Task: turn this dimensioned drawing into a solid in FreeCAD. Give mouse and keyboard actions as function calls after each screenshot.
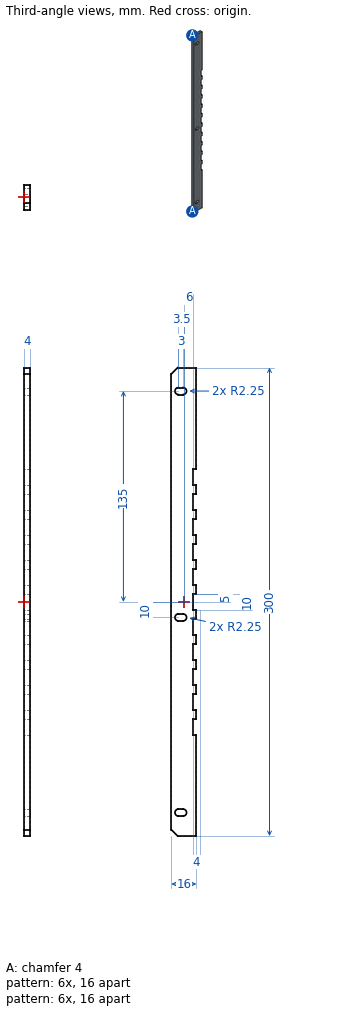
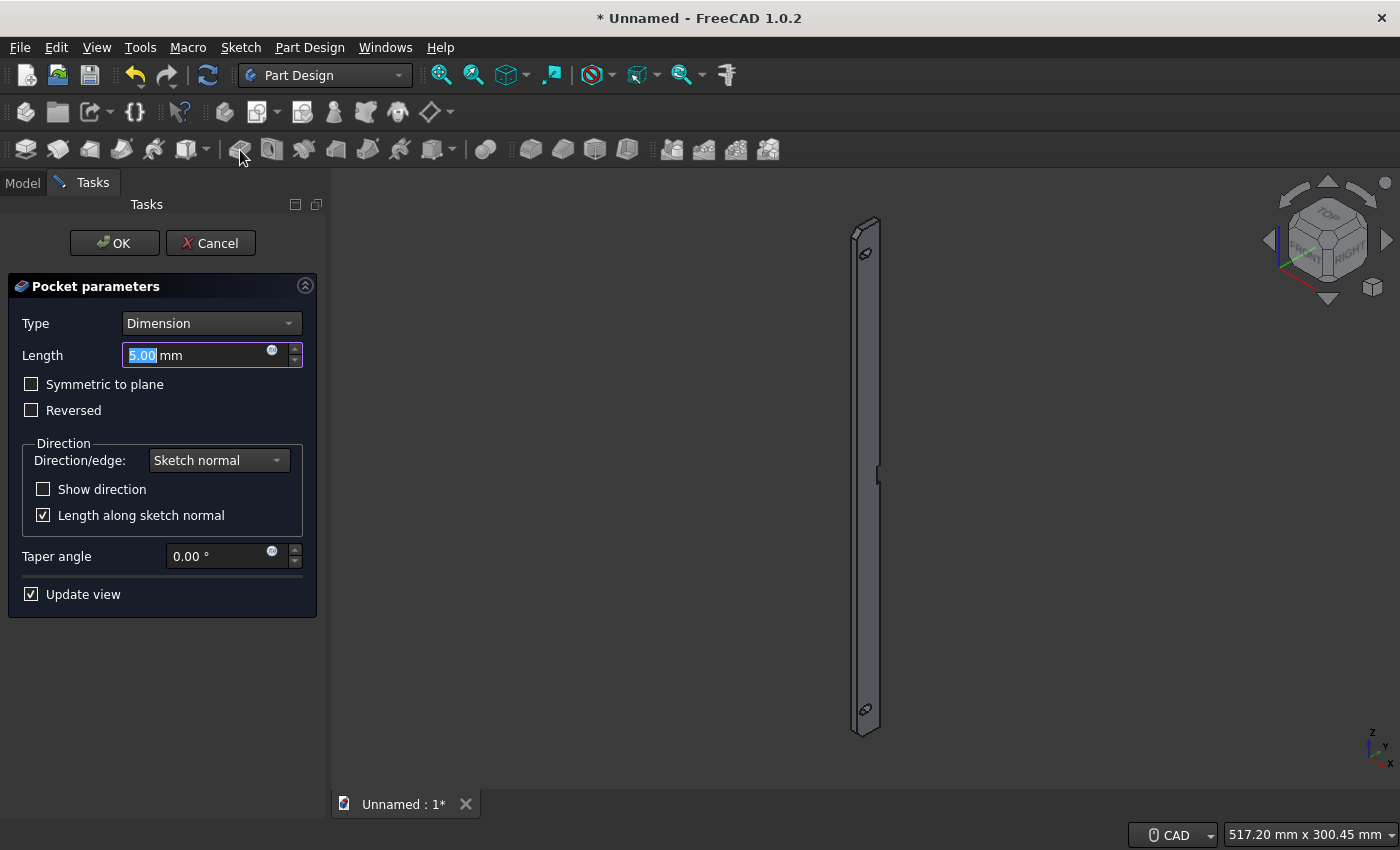
click(212, 324)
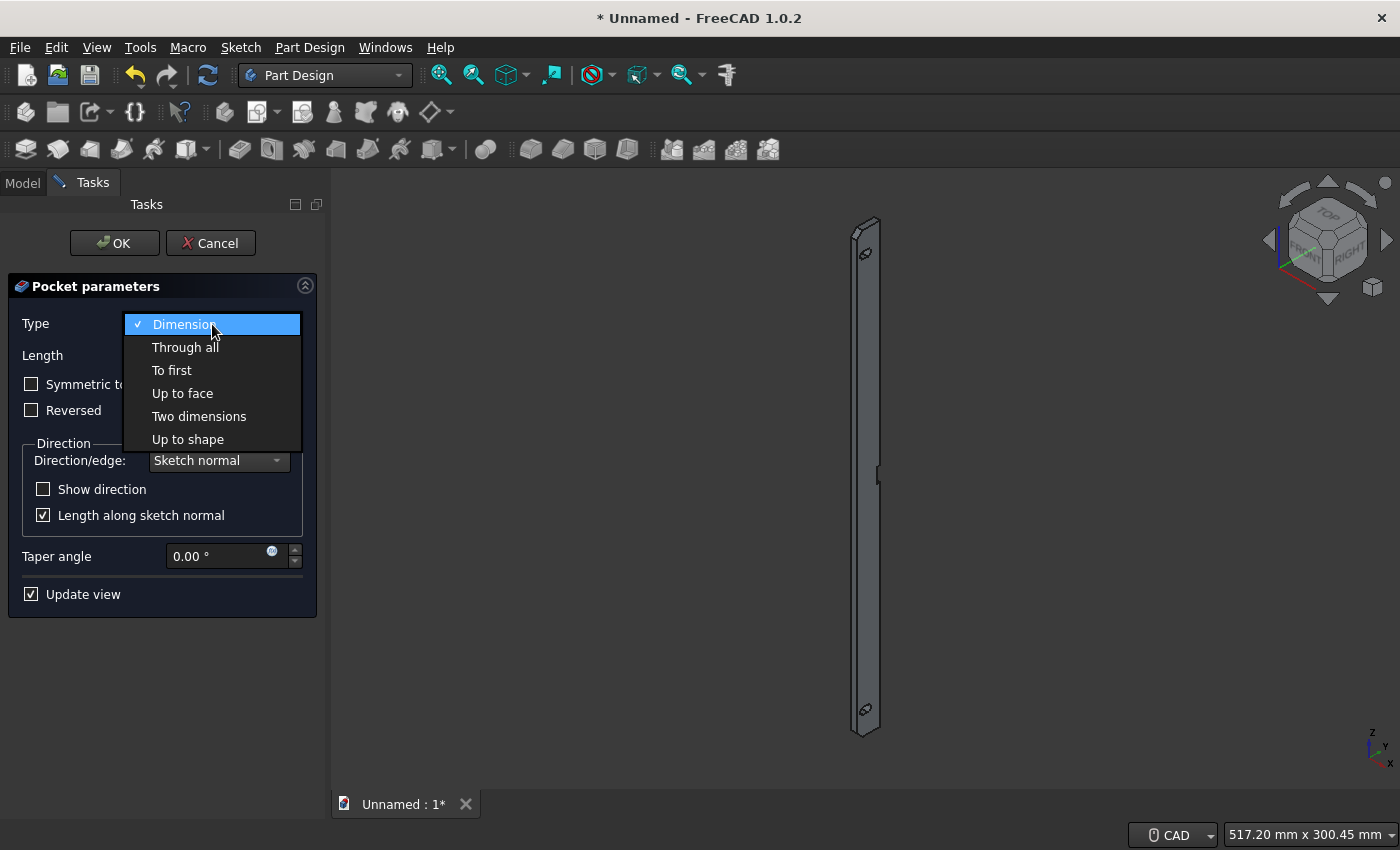
click(212, 348)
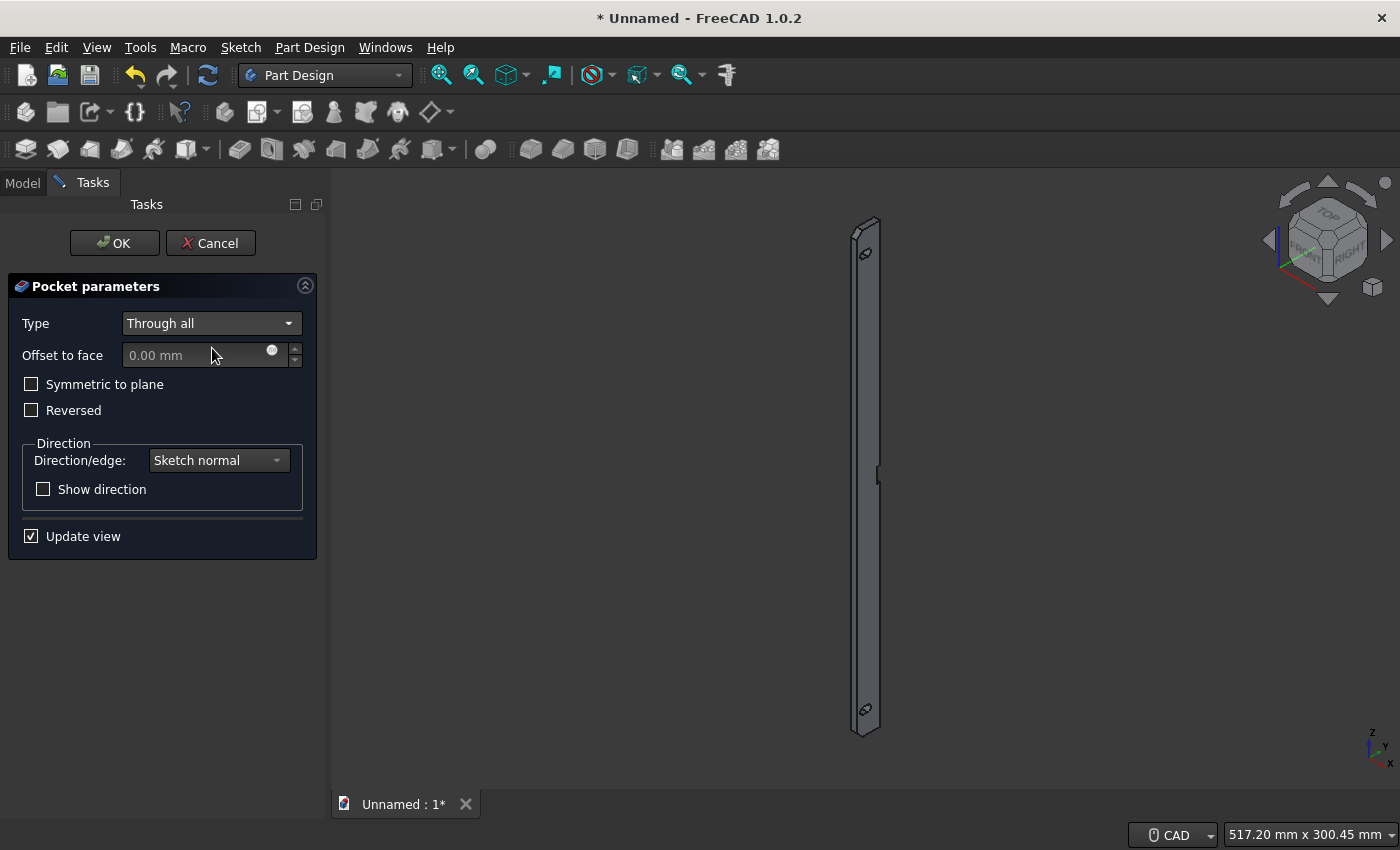
click(115, 243)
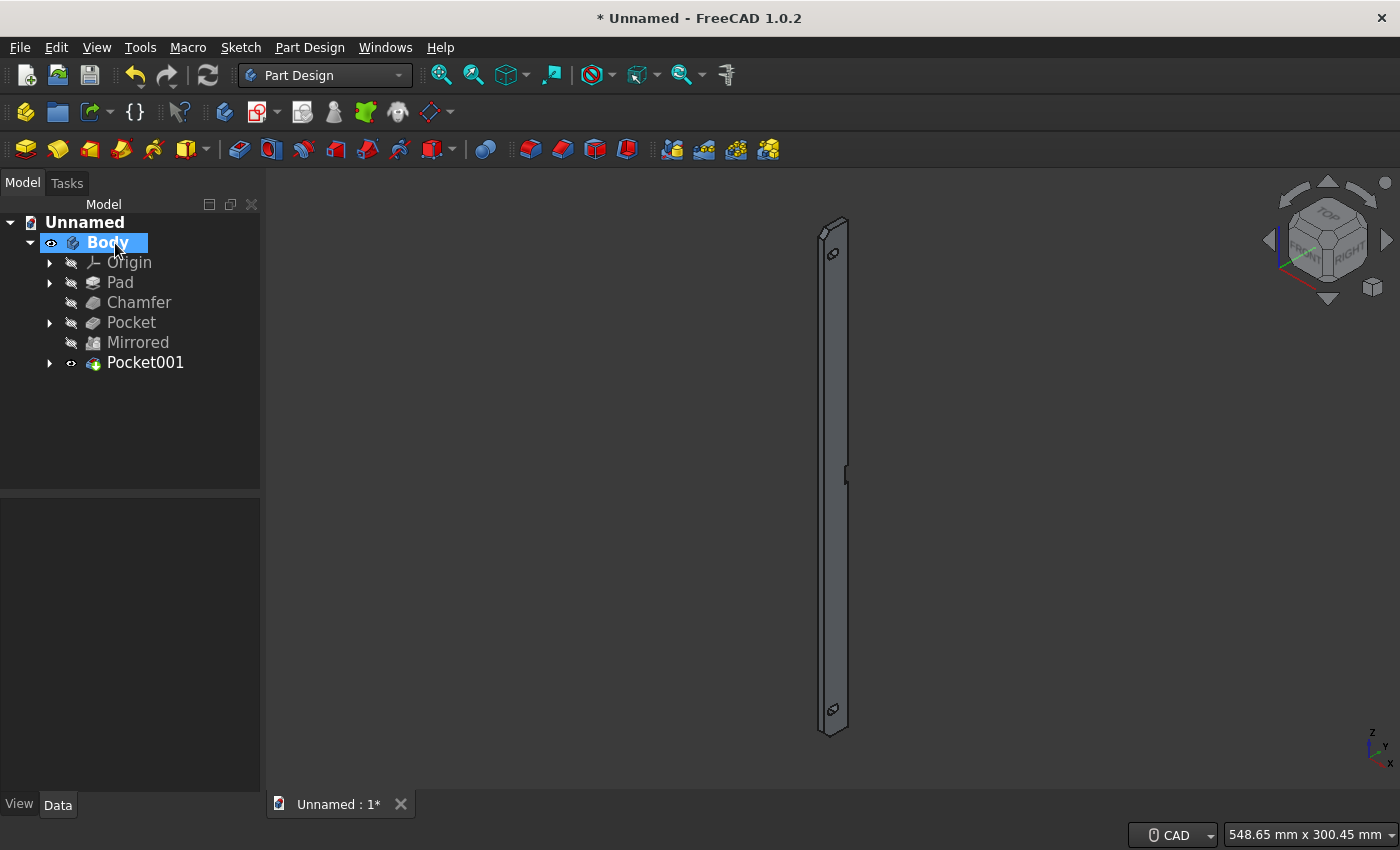
click(116, 363)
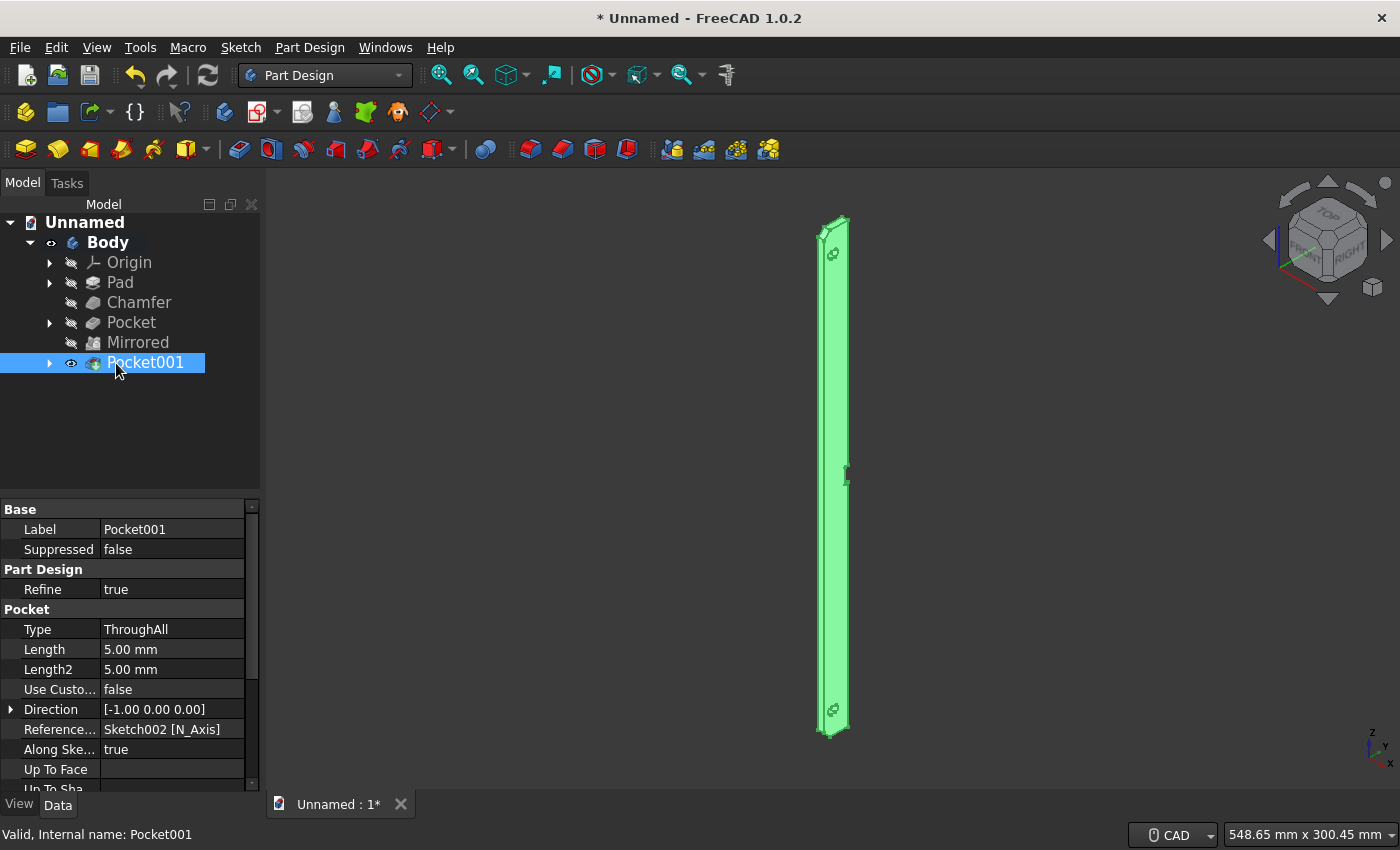
click(704, 150)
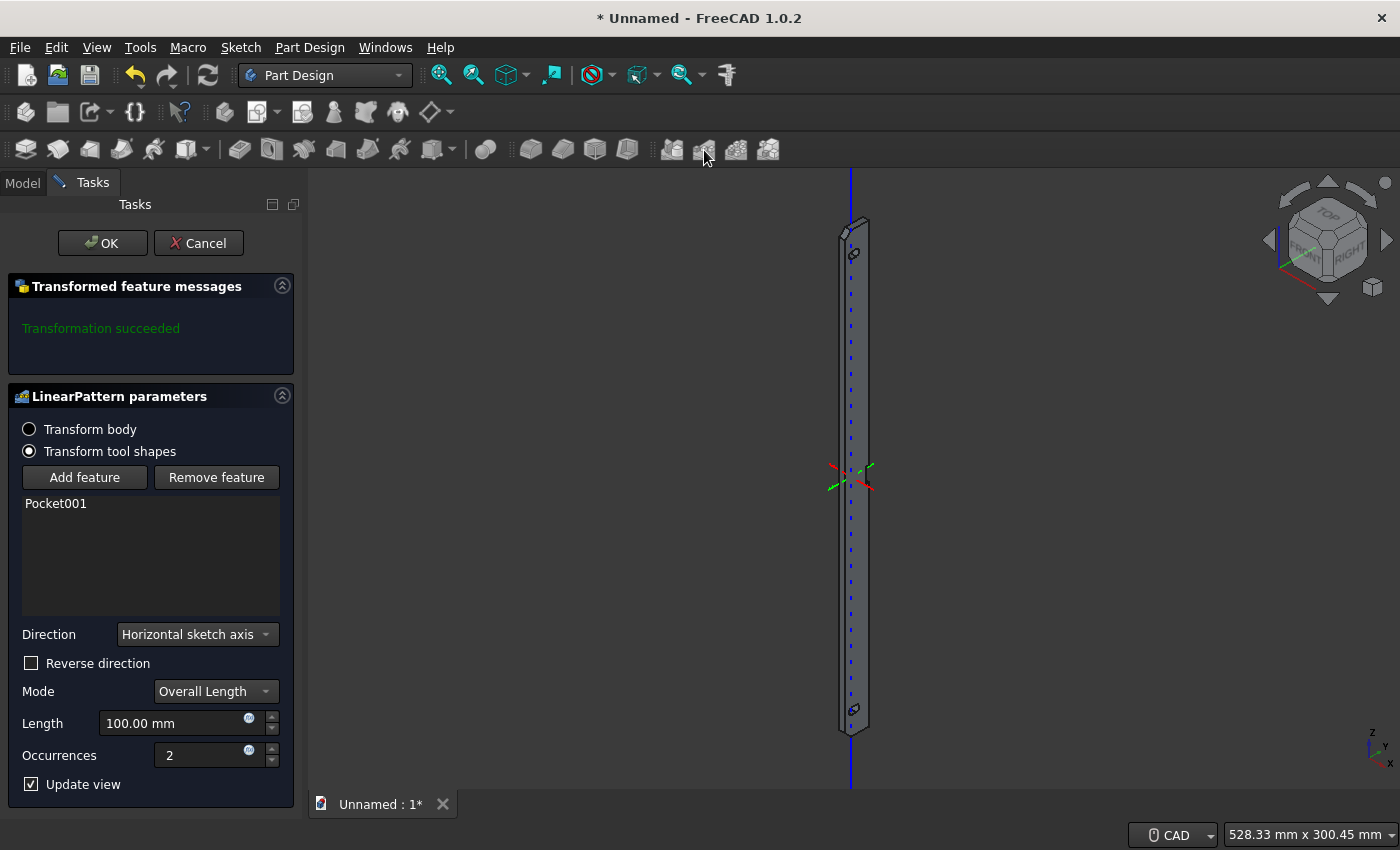
click(198, 634)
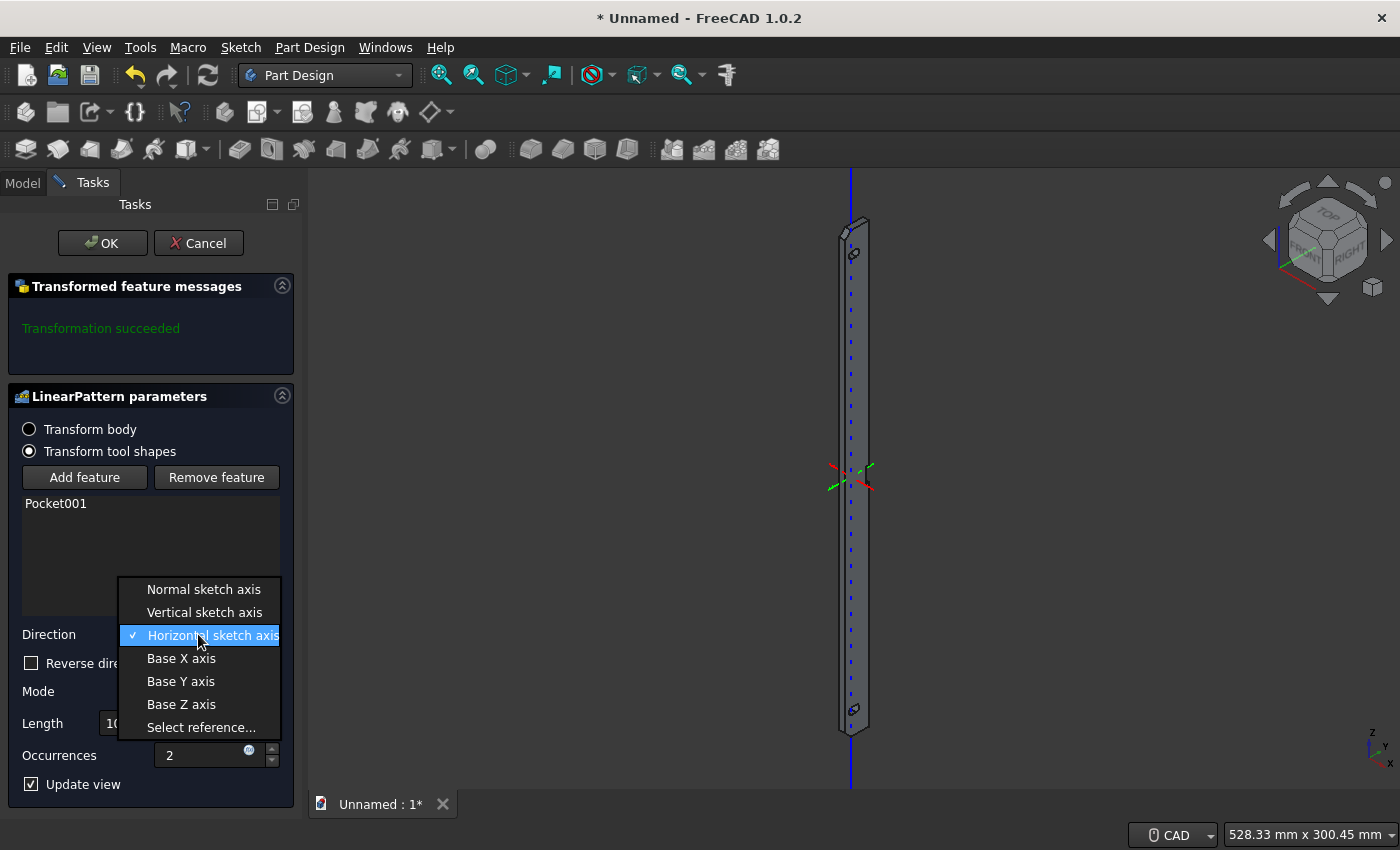
click(198, 704)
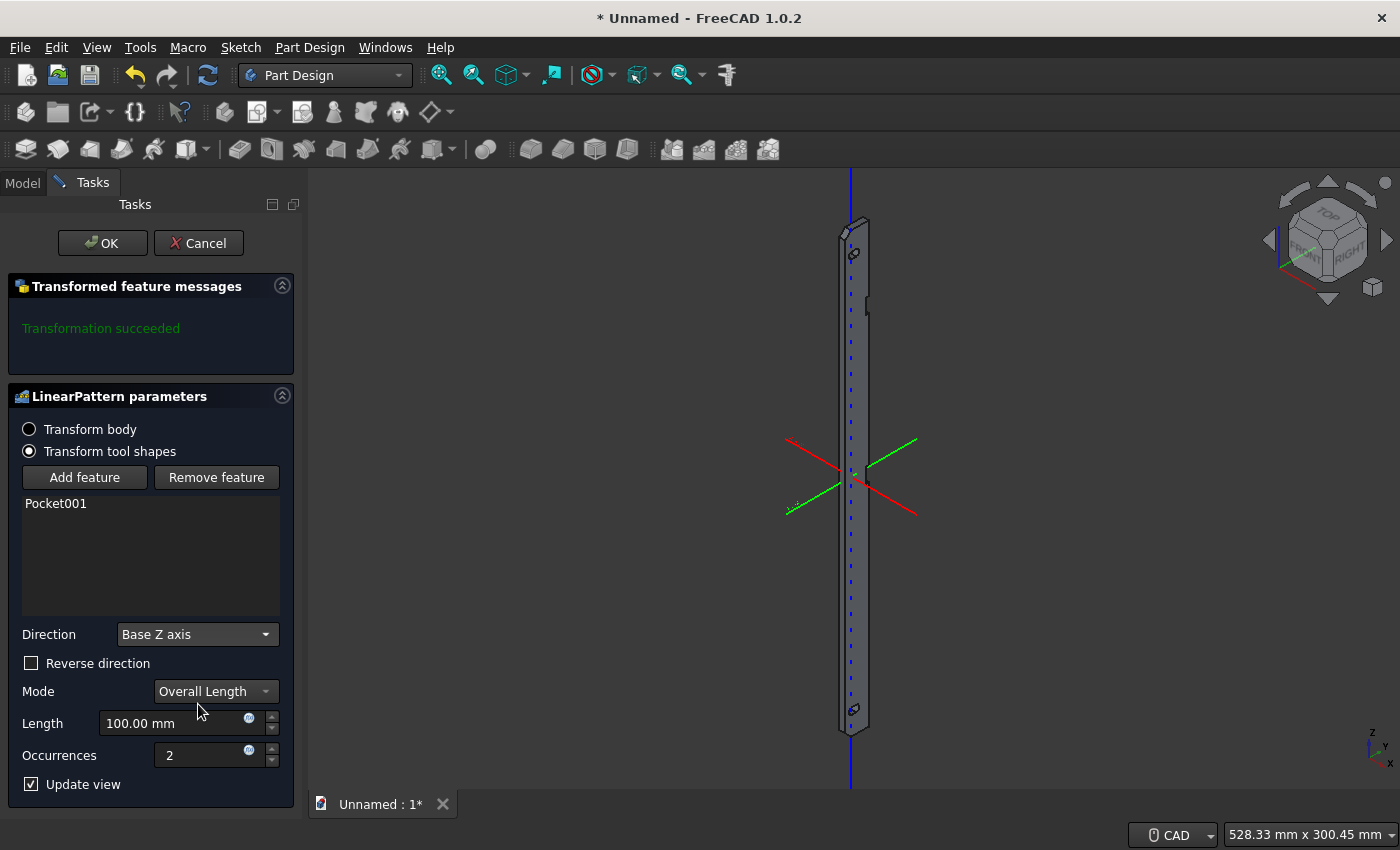
click(217, 692)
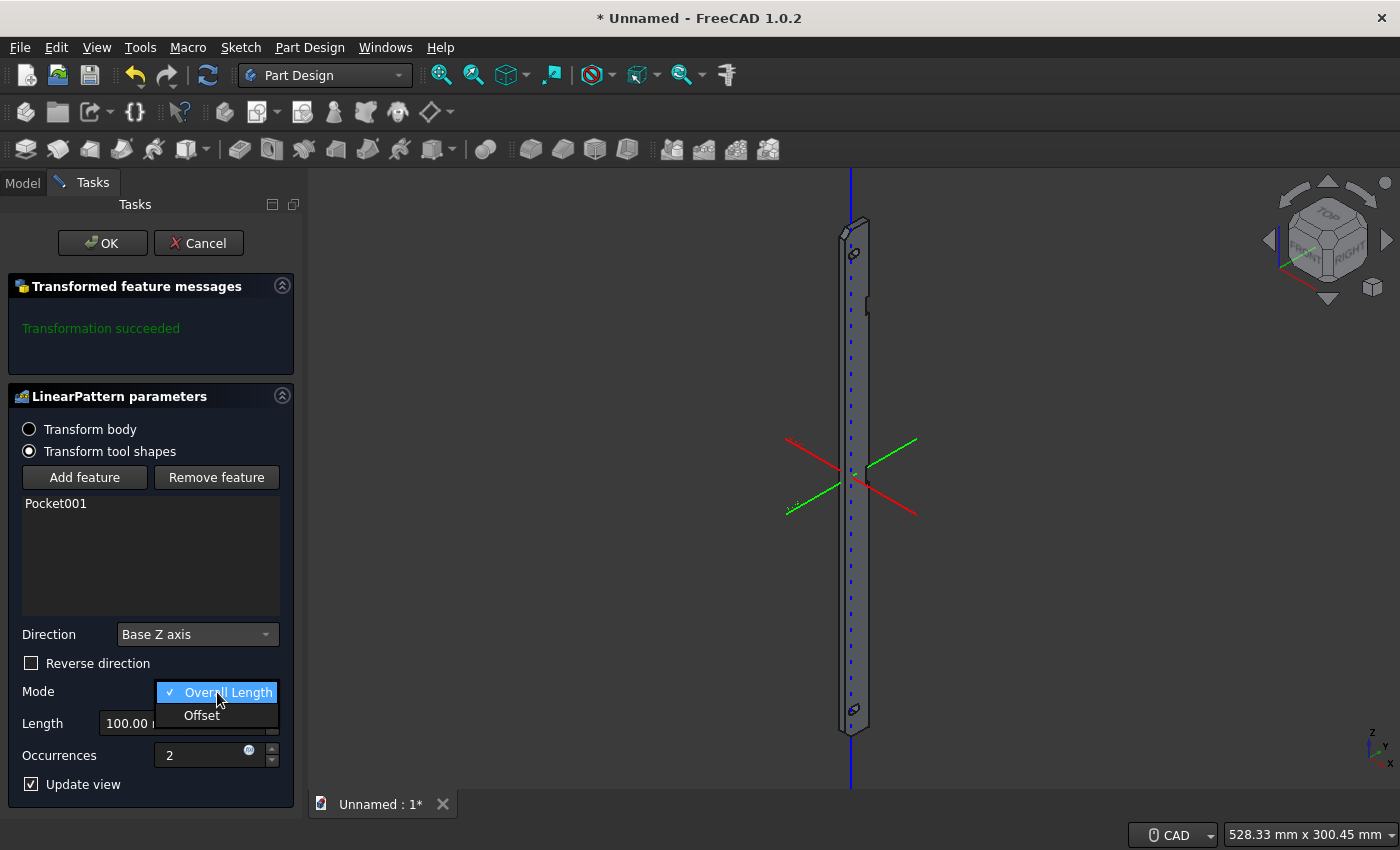
click(216, 716)